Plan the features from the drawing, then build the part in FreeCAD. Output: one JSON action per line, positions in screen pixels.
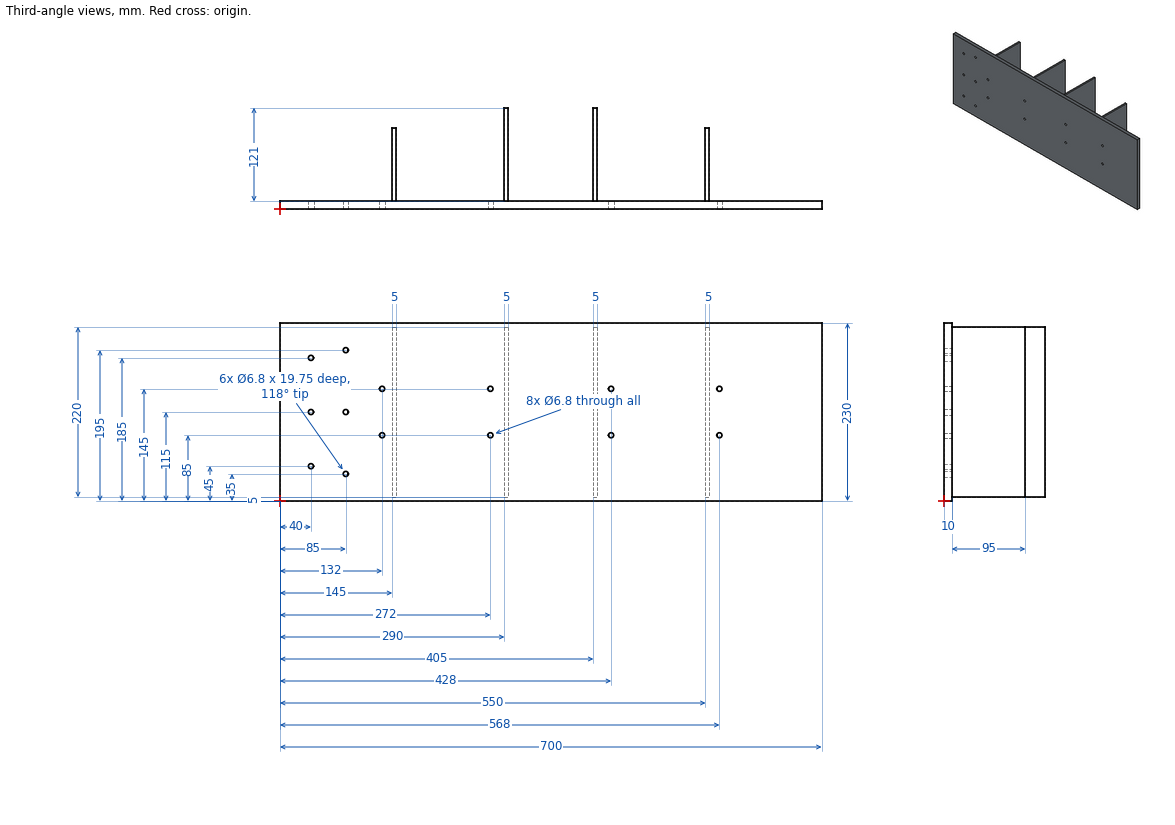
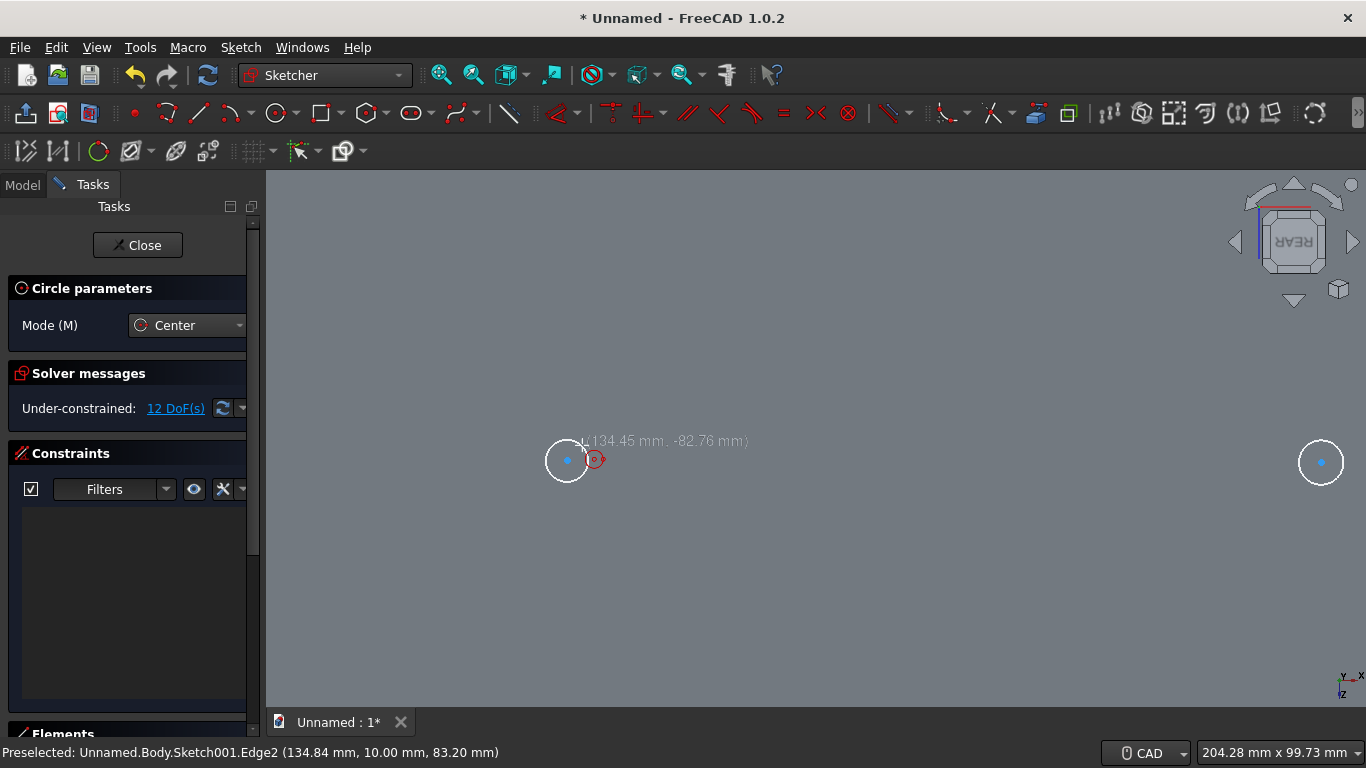
{"action": "scroll", "coordinate": [583, 448], "scroll_direction": "down", "scroll_amount": 8}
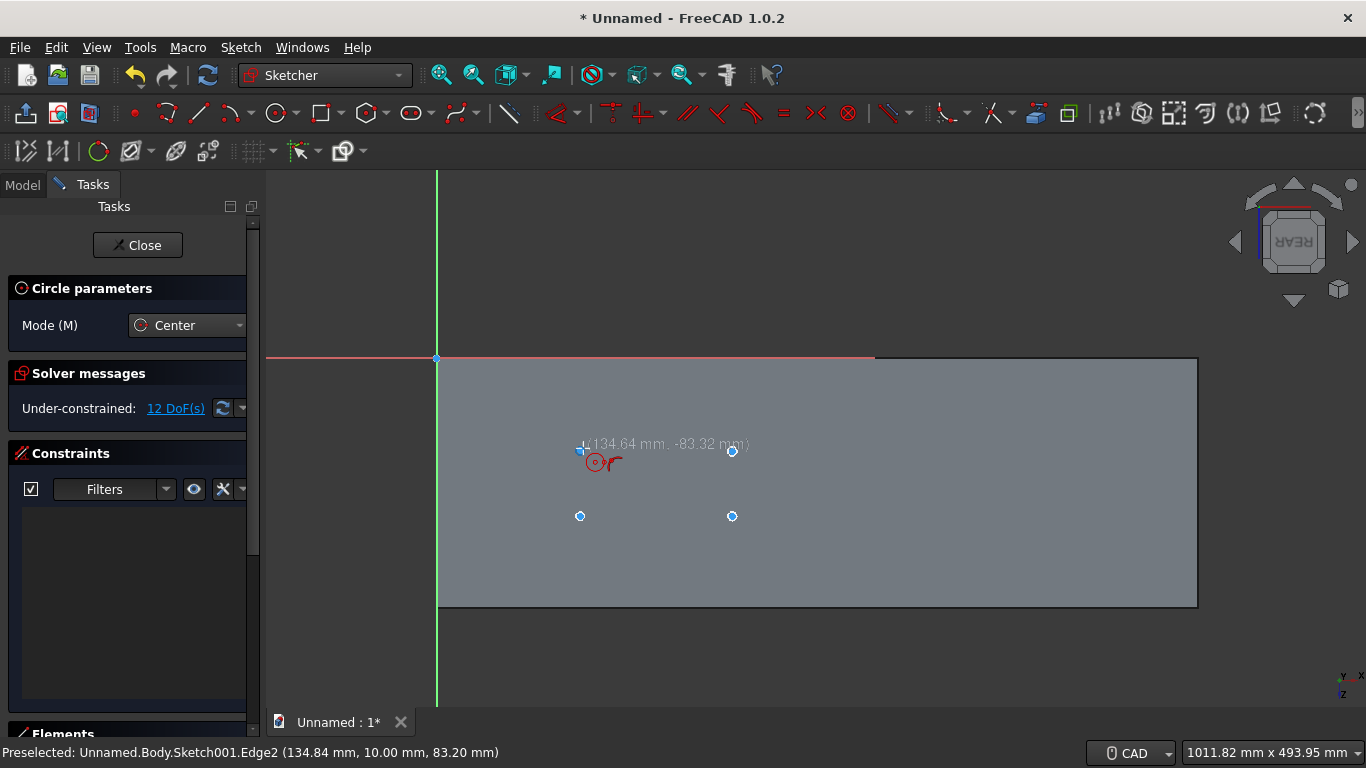
{"action": "scroll", "coordinate": [1054, 450], "scroll_direction": "up", "scroll_amount": 10}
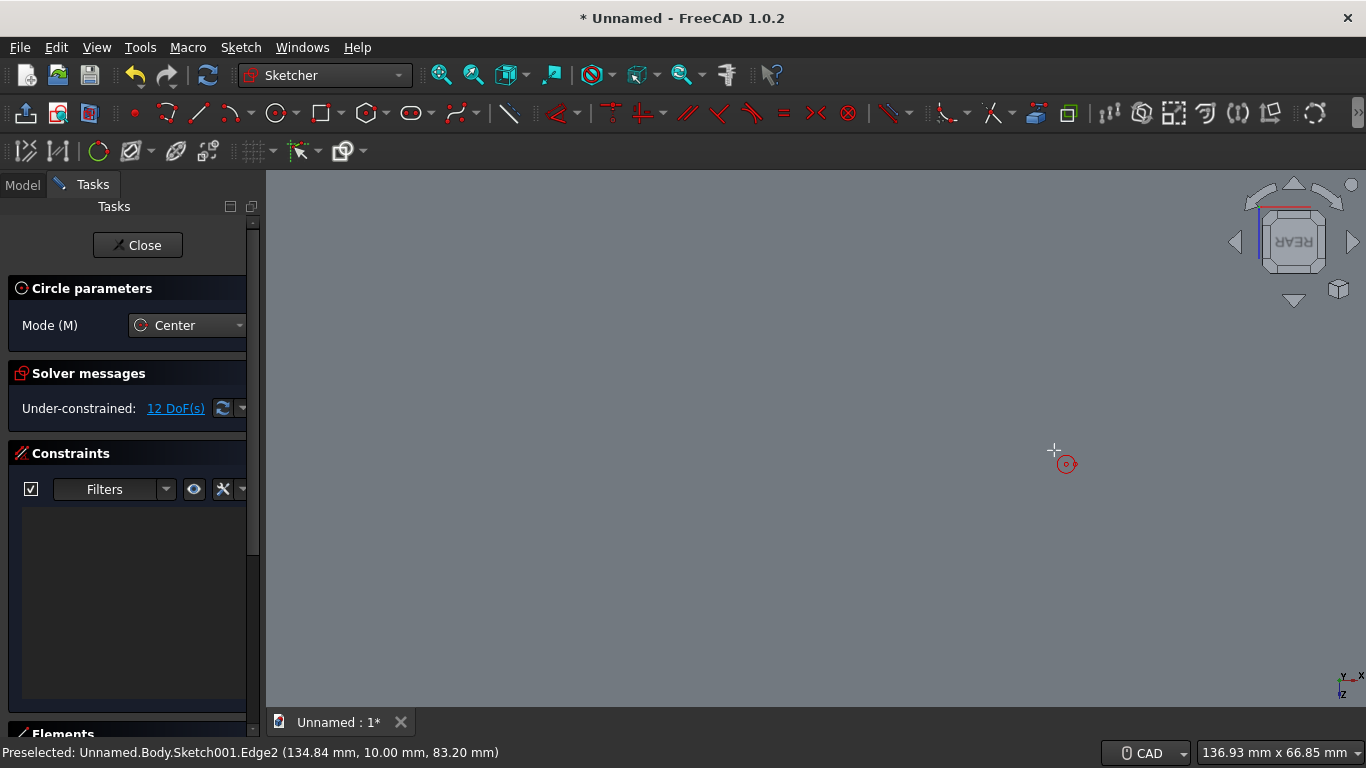
{"action": "scroll", "coordinate": [1055, 450], "scroll_direction": "down", "scroll_amount": 10}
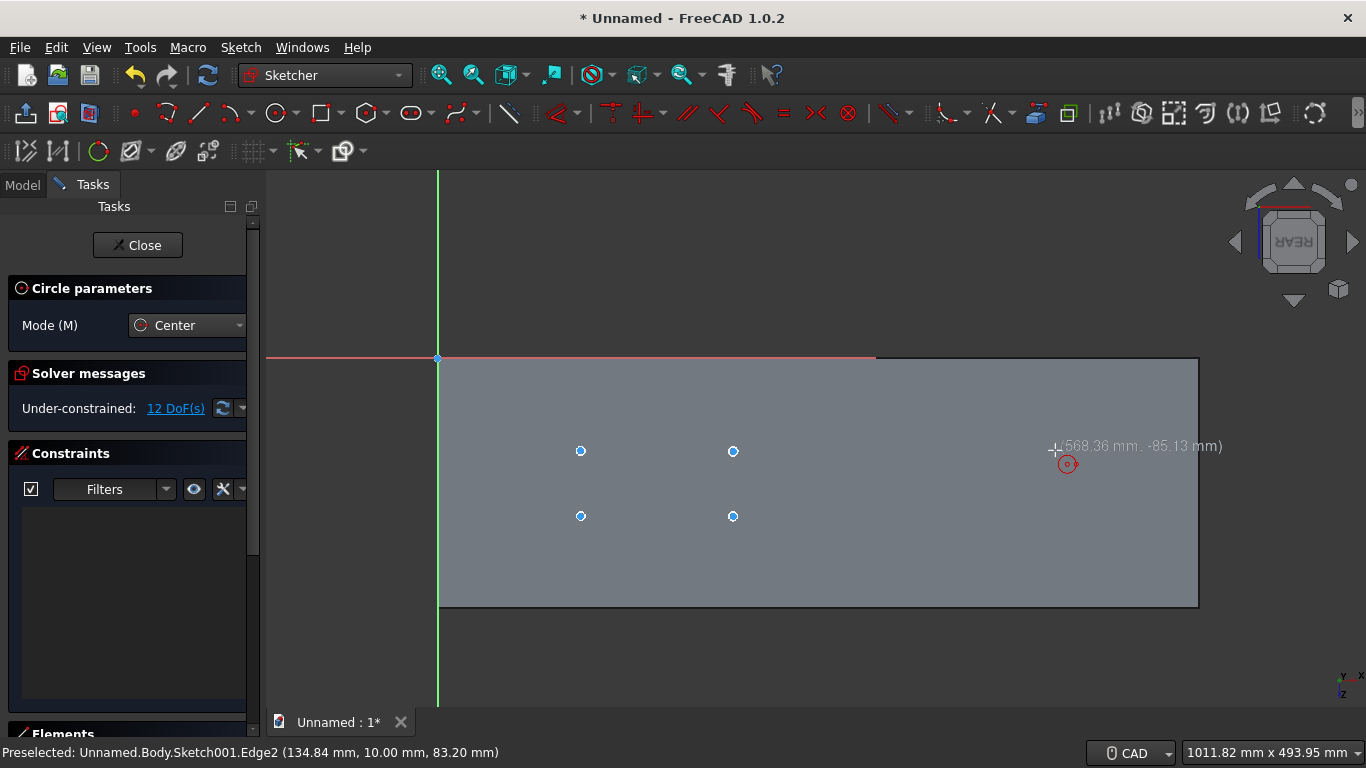
{"action": "left_click", "coordinate": [1055, 450]}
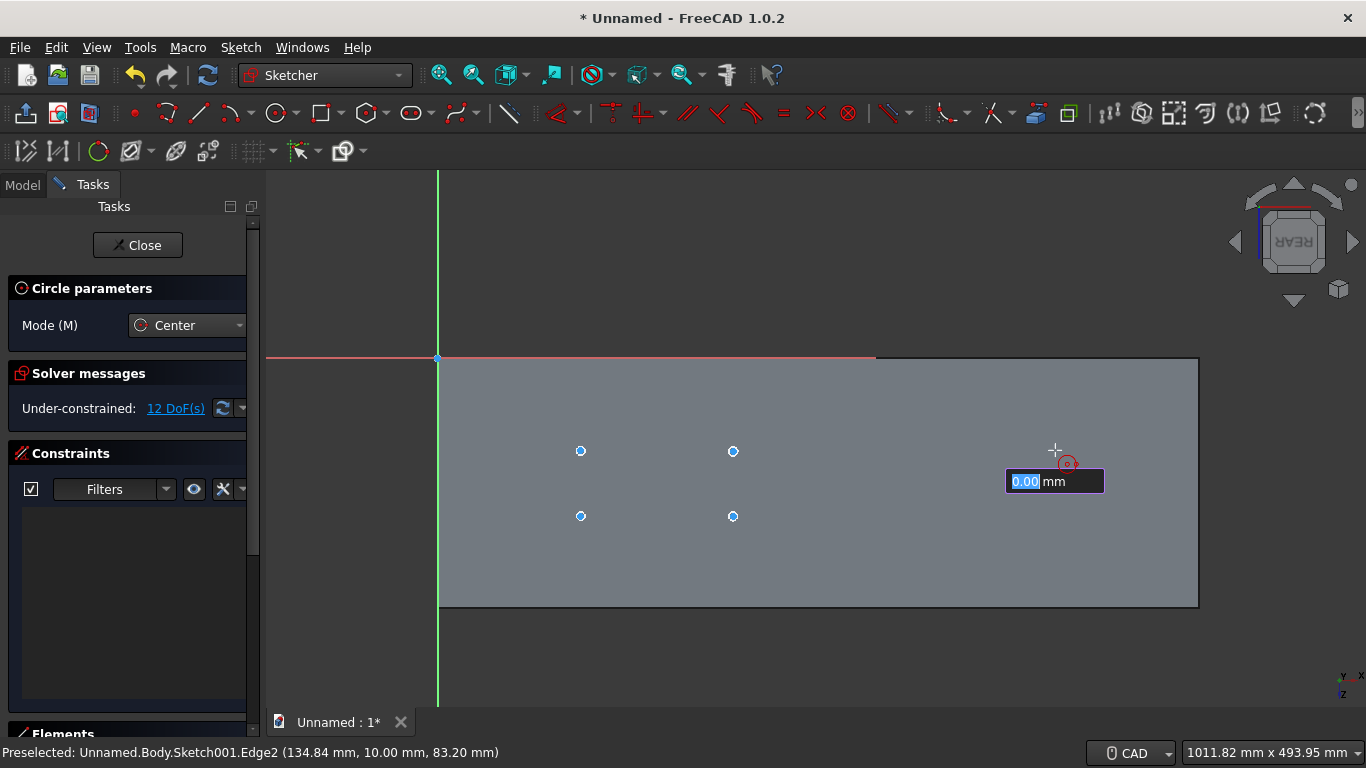
{"action": "scroll", "coordinate": [1058, 448], "scroll_direction": "up", "scroll_amount": 8}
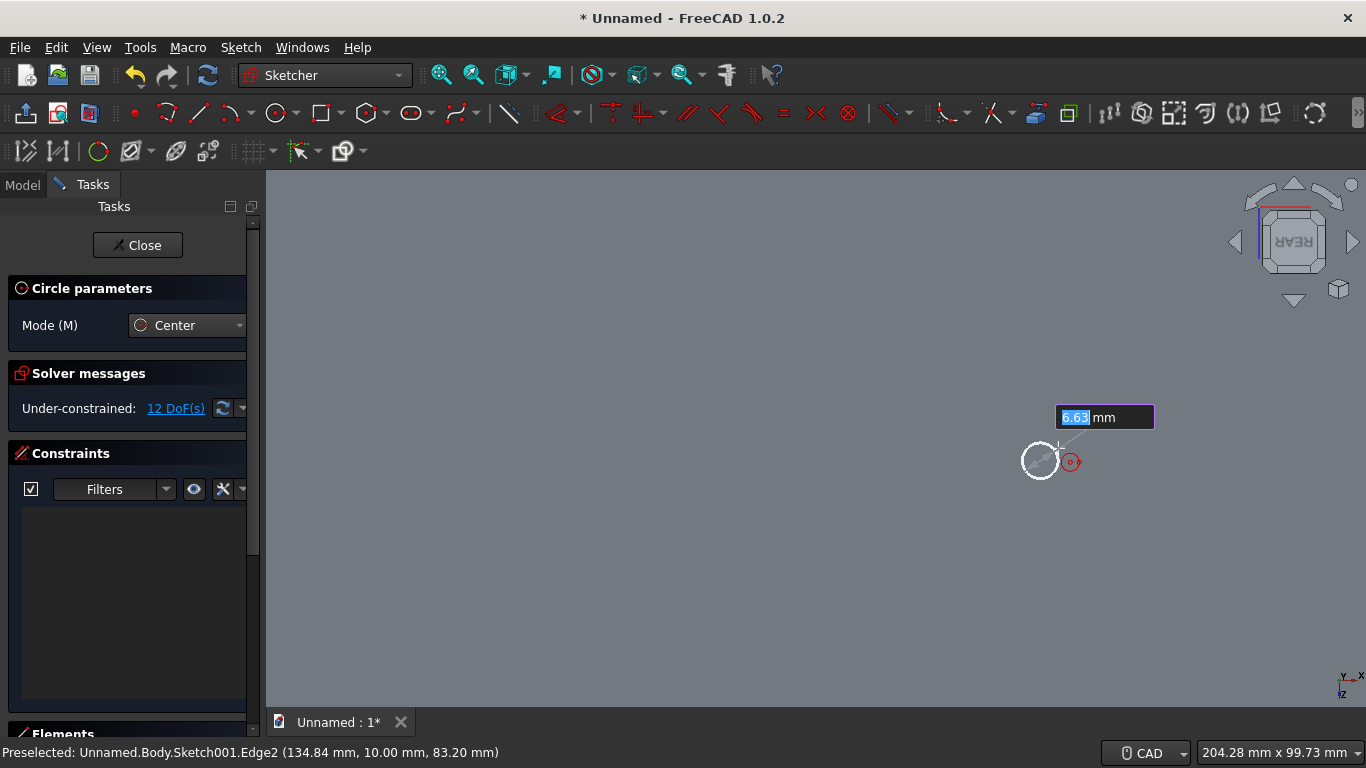
{"action": "left_click", "coordinate": [1054, 445]}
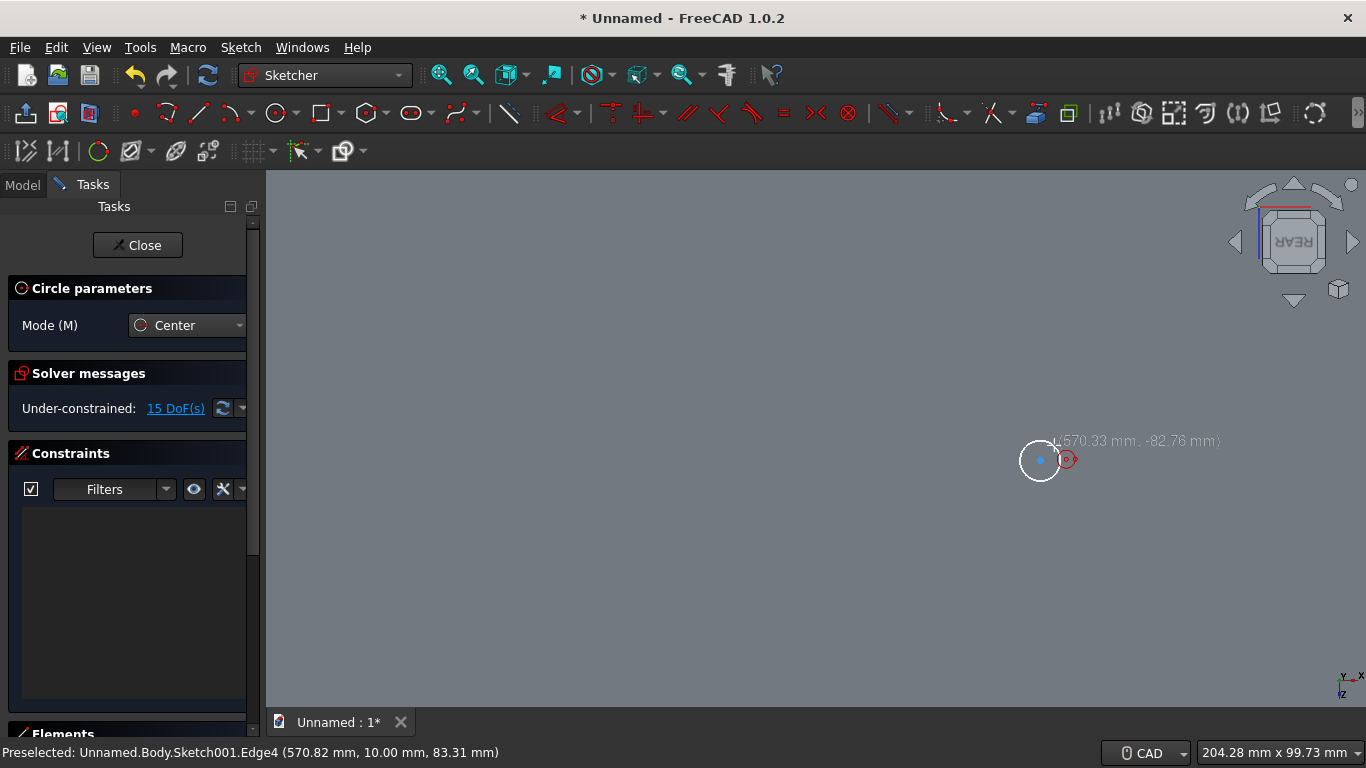
{"action": "scroll", "coordinate": [1058, 448], "scroll_direction": "down", "scroll_amount": 8}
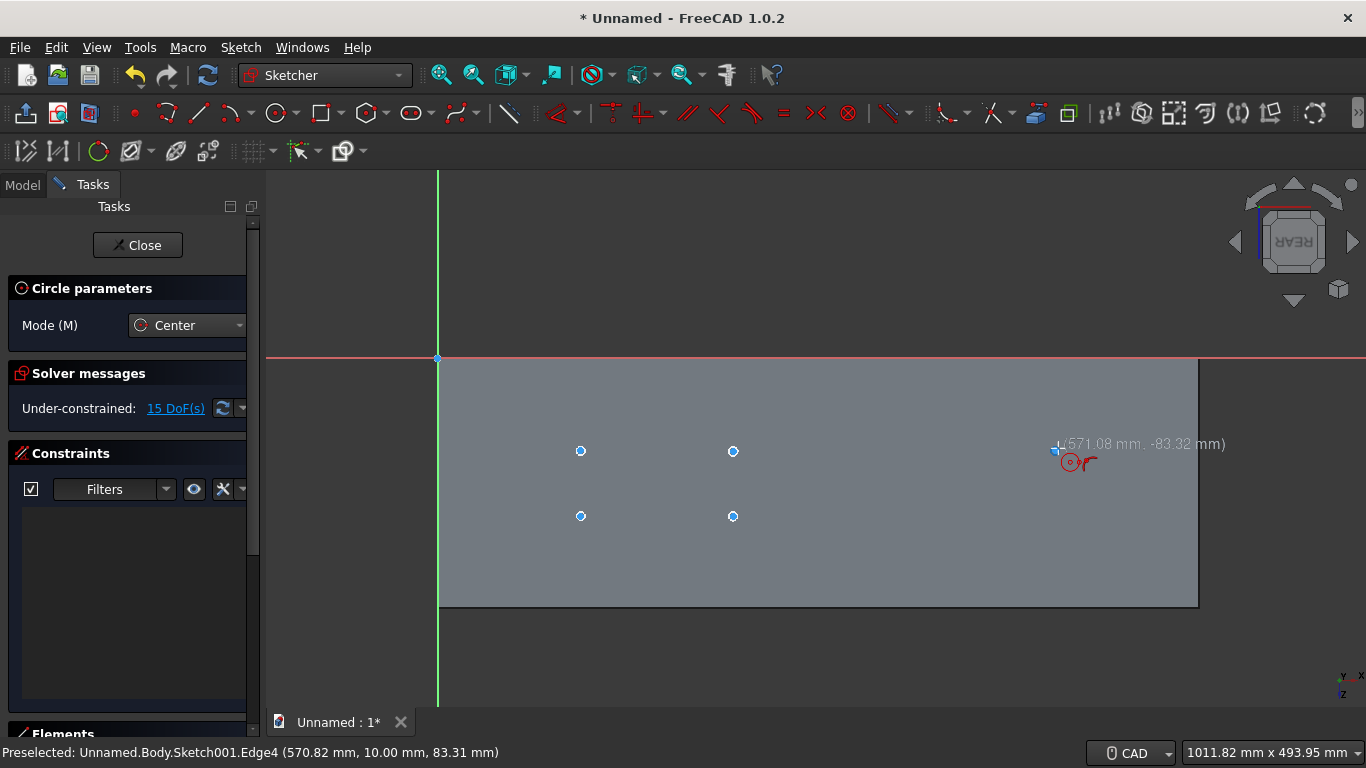
{"action": "scroll", "coordinate": [1055, 516], "scroll_direction": "up", "scroll_amount": 10}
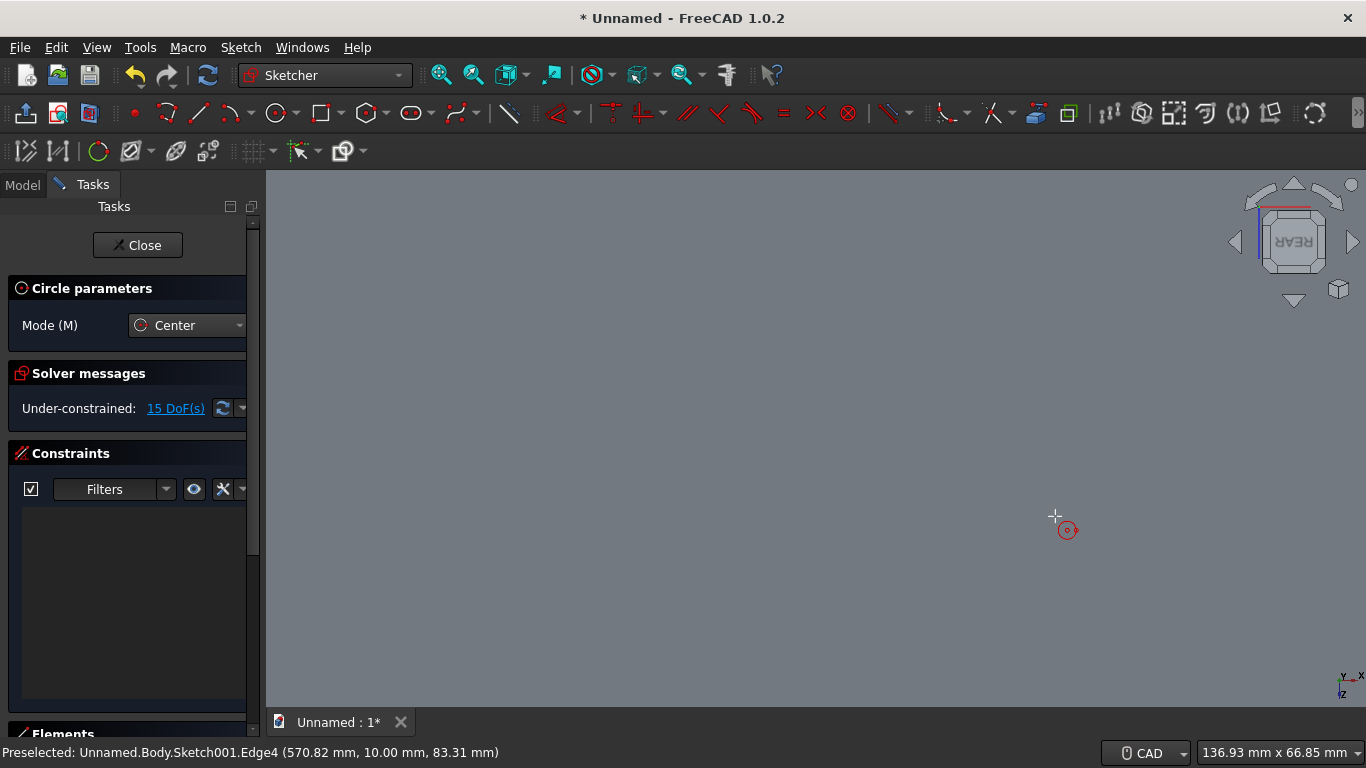
{"action": "scroll", "coordinate": [1055, 516], "scroll_direction": "down", "scroll_amount": 10}